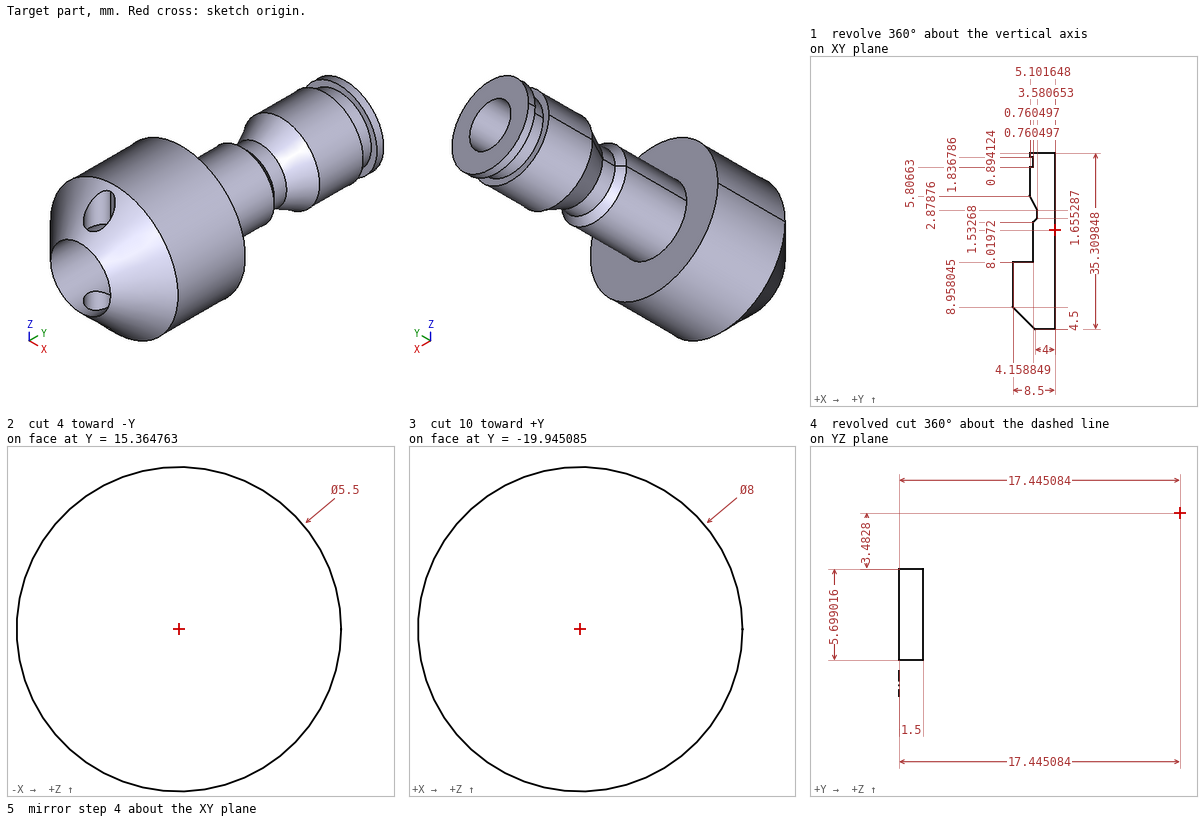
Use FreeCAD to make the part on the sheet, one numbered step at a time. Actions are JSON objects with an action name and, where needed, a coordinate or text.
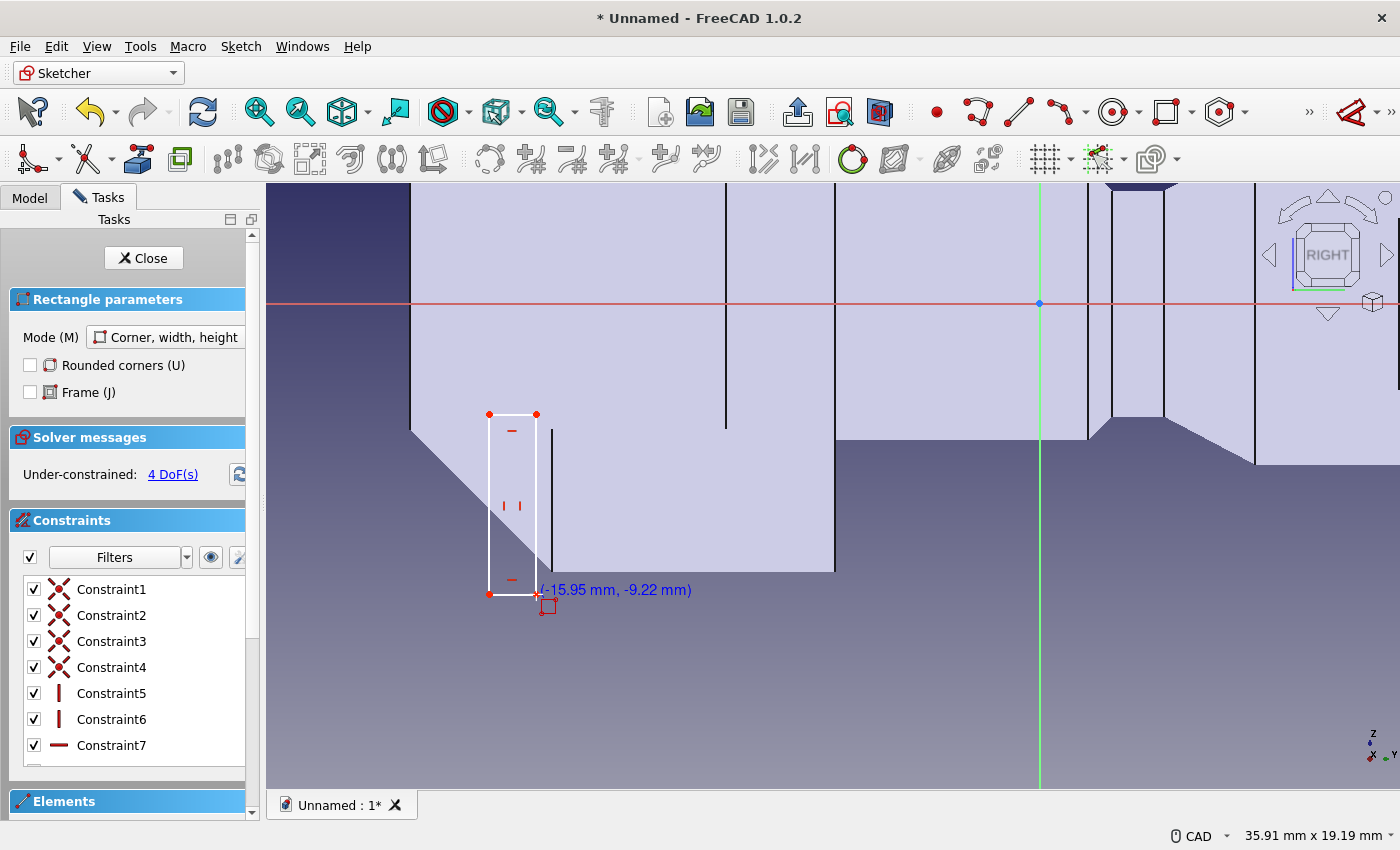
{"action": "left_click", "coordinate": [1019, 112]}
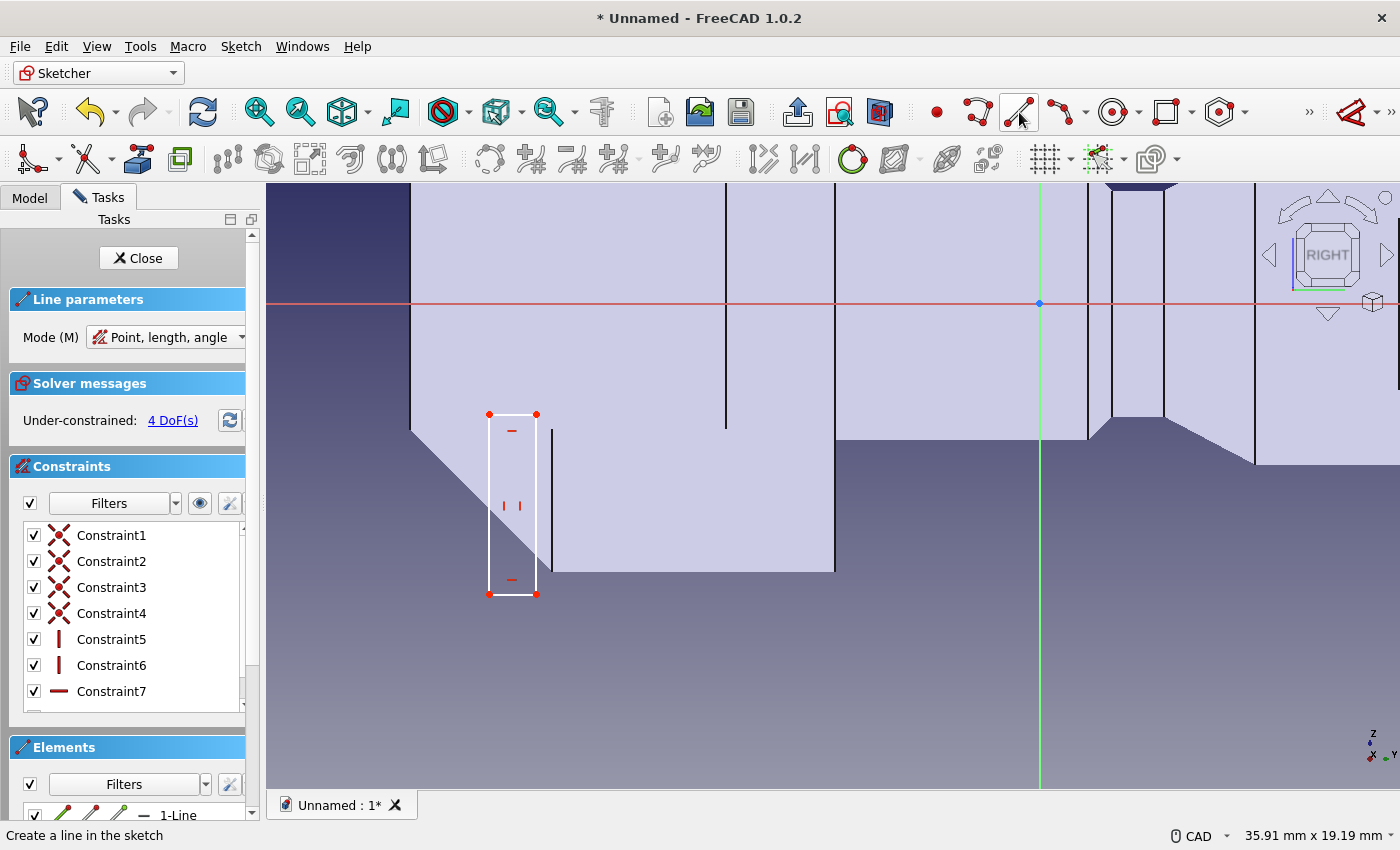
{"action": "left_click", "coordinate": [489, 612]}
{"action": "left_click", "coordinate": [489, 666]}
{"action": "key", "text": "Escape"}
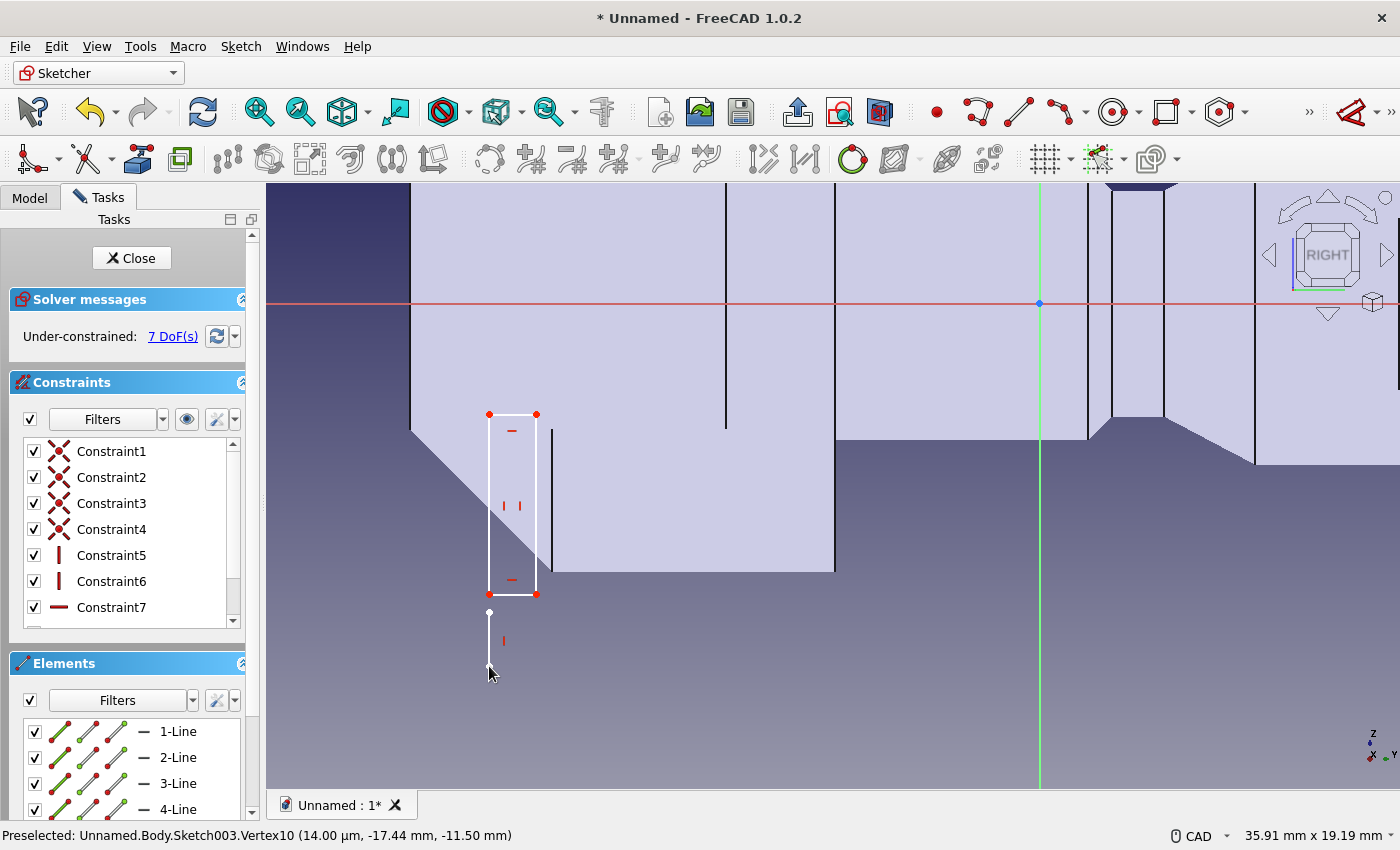
{"action": "left_click", "coordinate": [489, 629]}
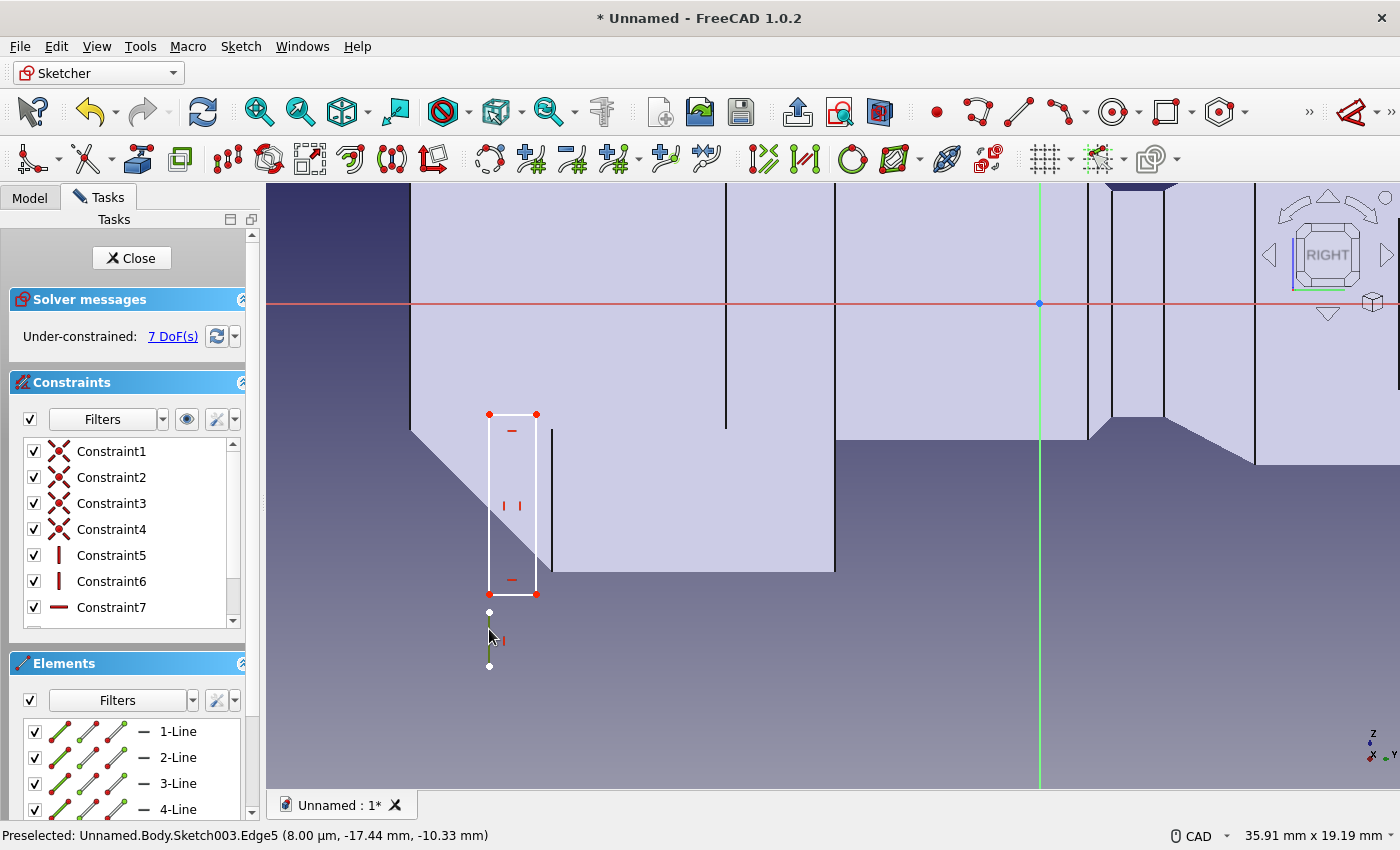
{"action": "key", "text": "g n"}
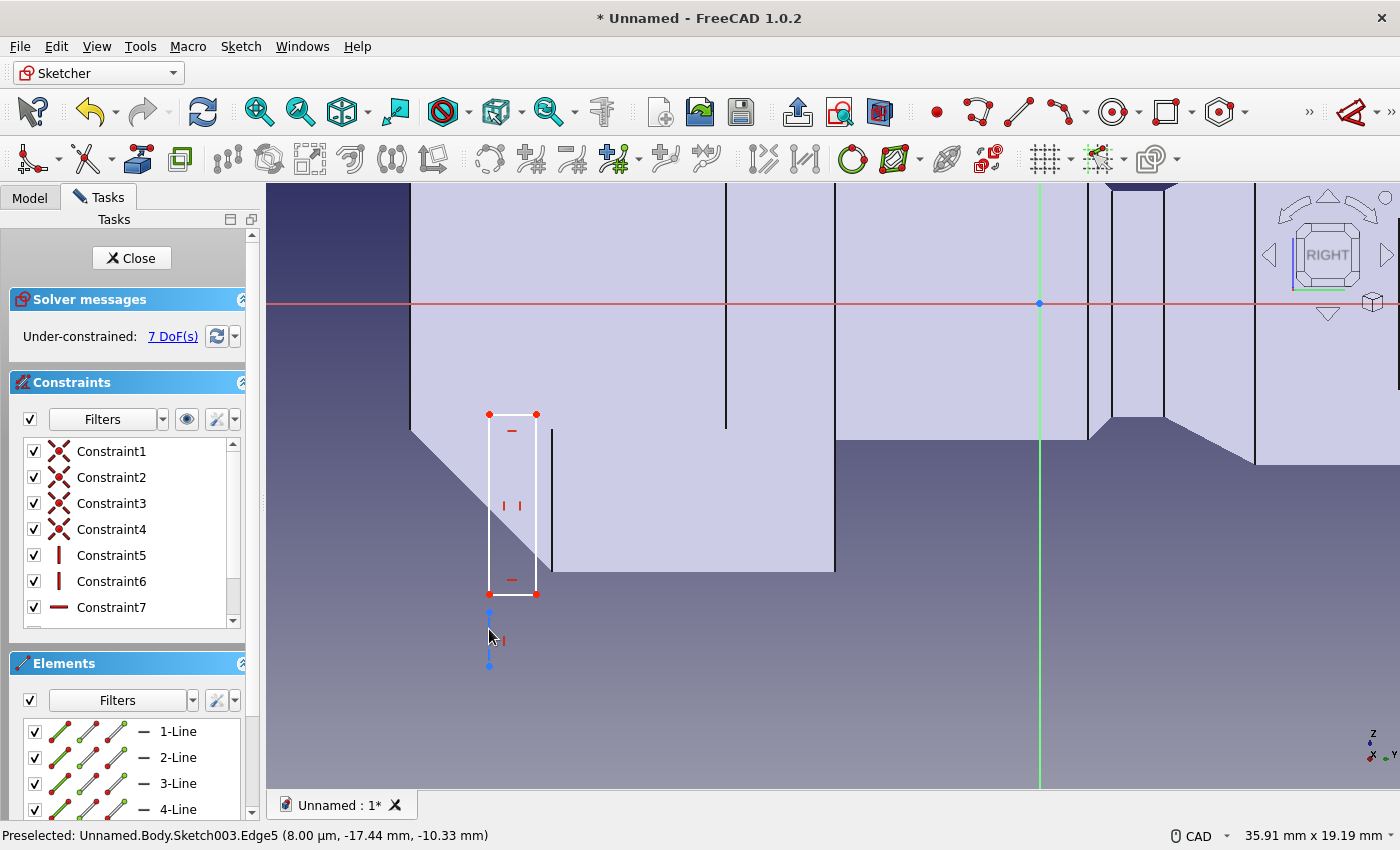
{"action": "left_click", "coordinate": [1350, 112]}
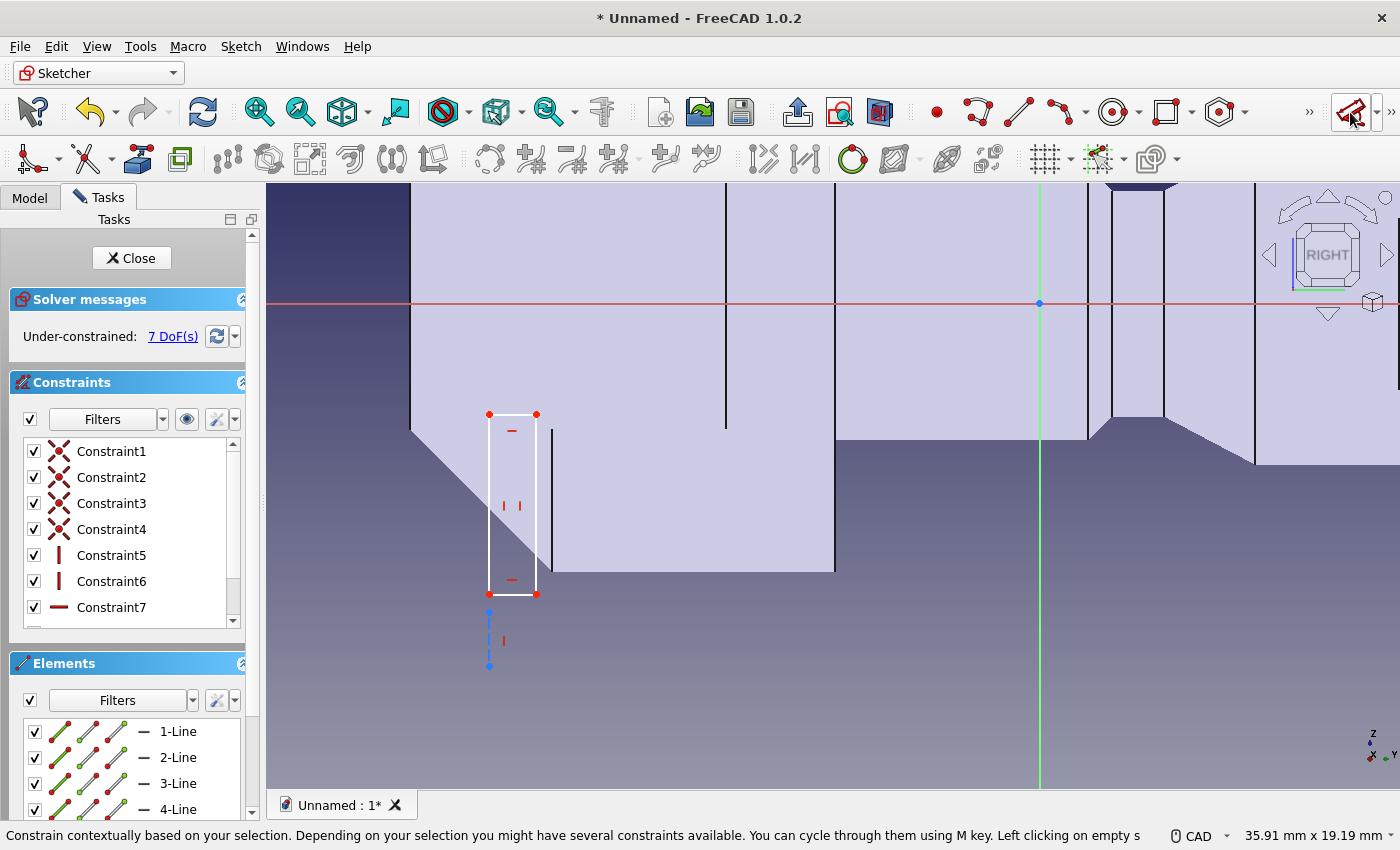
{"action": "left_click", "coordinate": [503, 595]}
{"action": "left_click", "coordinate": [512, 629]}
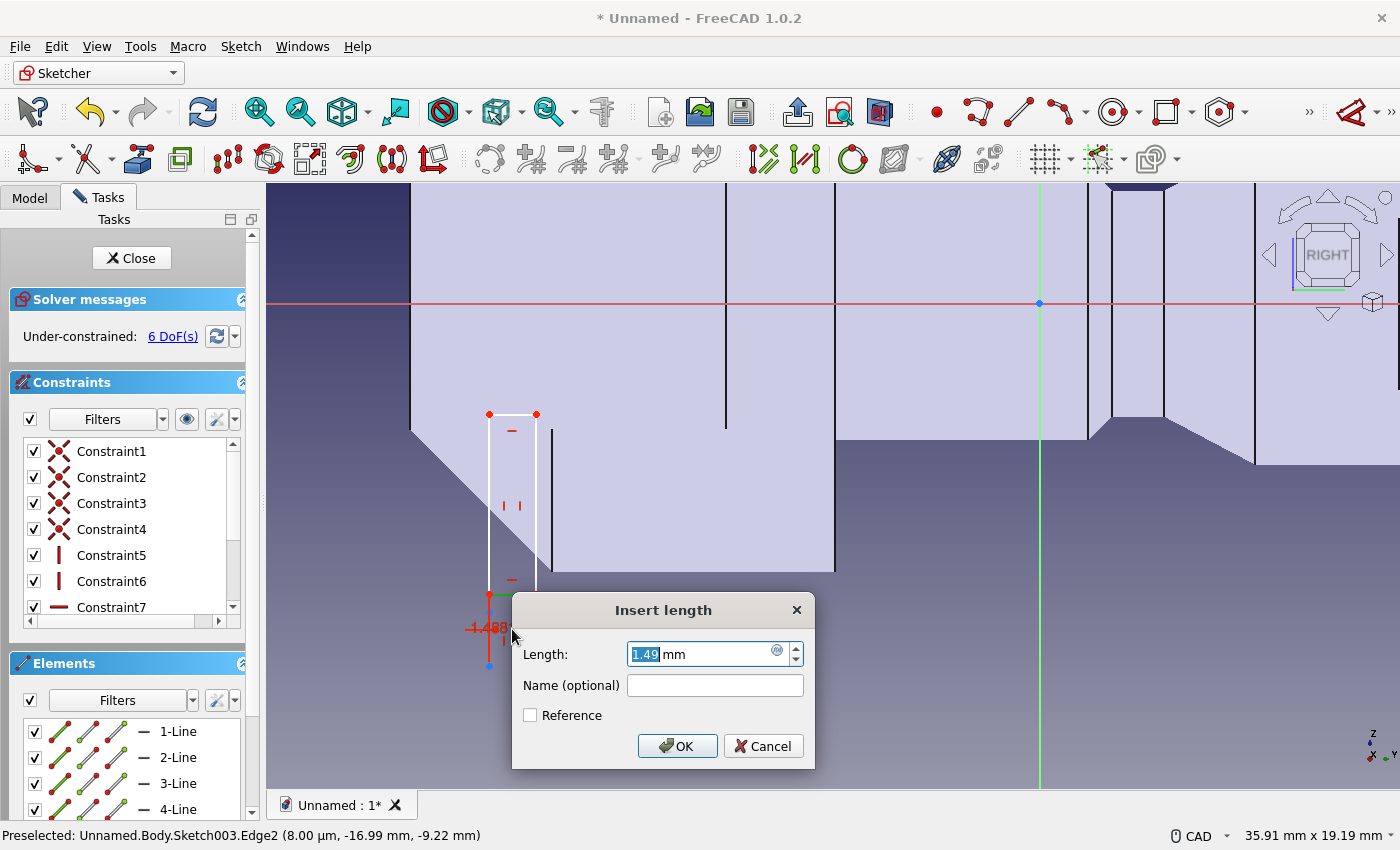
{"action": "type", "text": "1.5"}
{"action": "key", "text": "Return"}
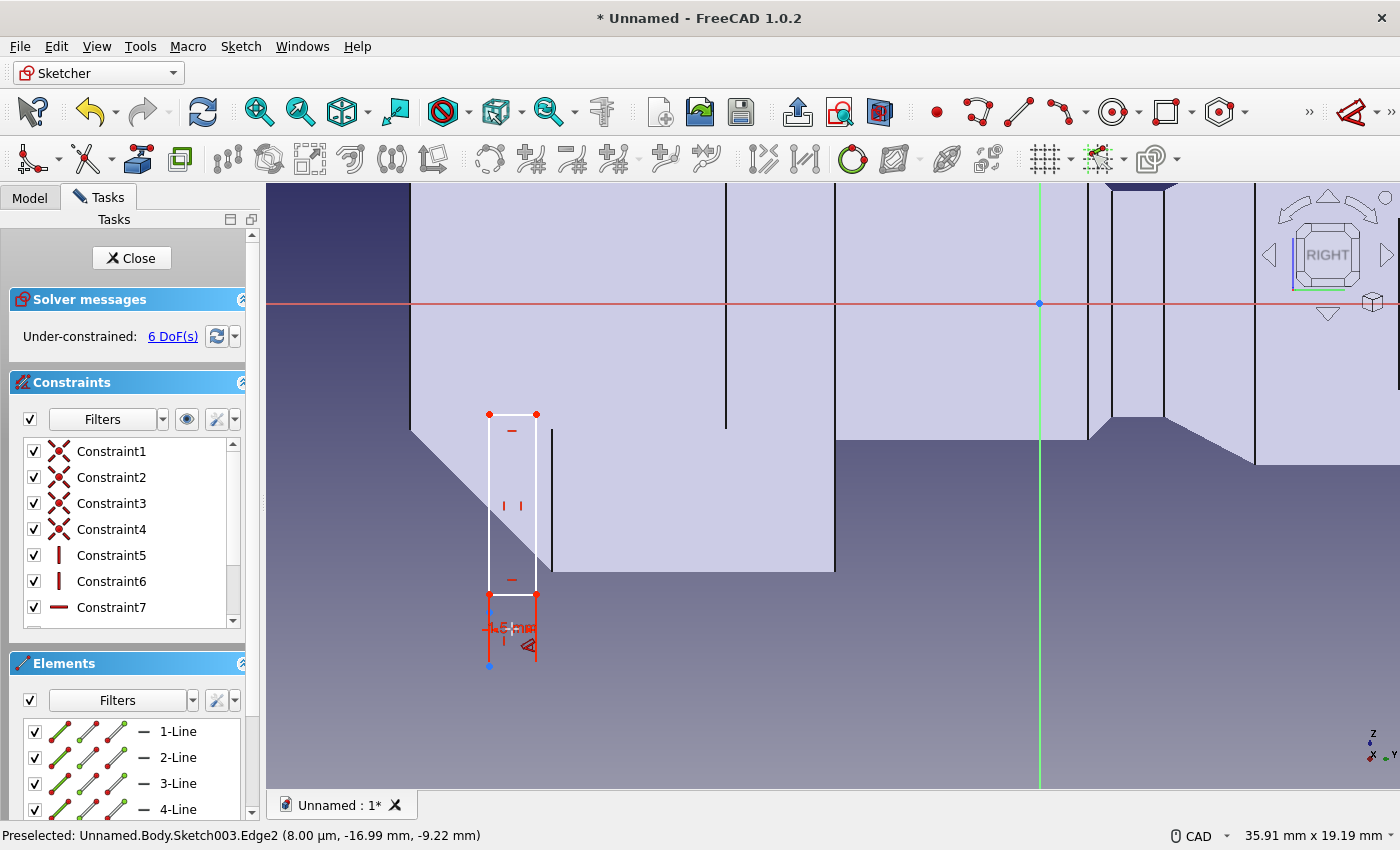
{"action": "left_click", "coordinate": [489, 415]}
{"action": "left_click", "coordinate": [1074, 359]}